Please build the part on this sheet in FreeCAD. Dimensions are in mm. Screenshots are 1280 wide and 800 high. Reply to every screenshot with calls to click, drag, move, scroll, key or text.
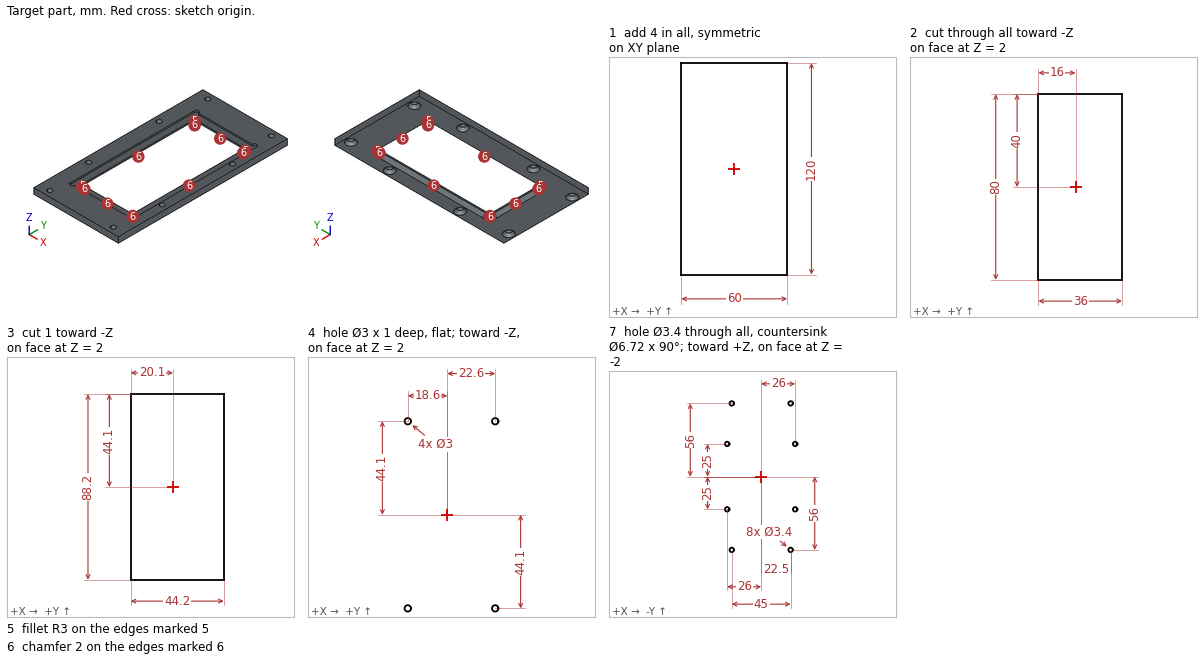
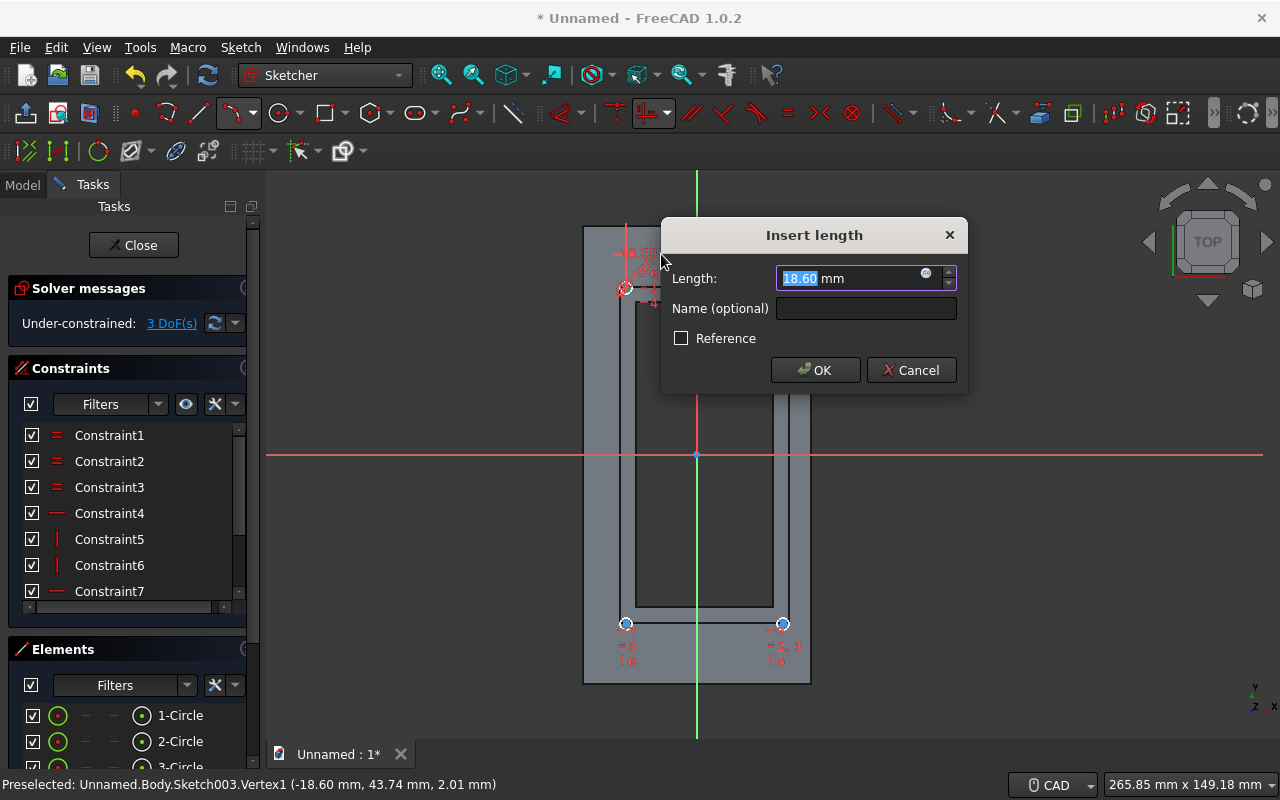
text(18.6)
key(Return)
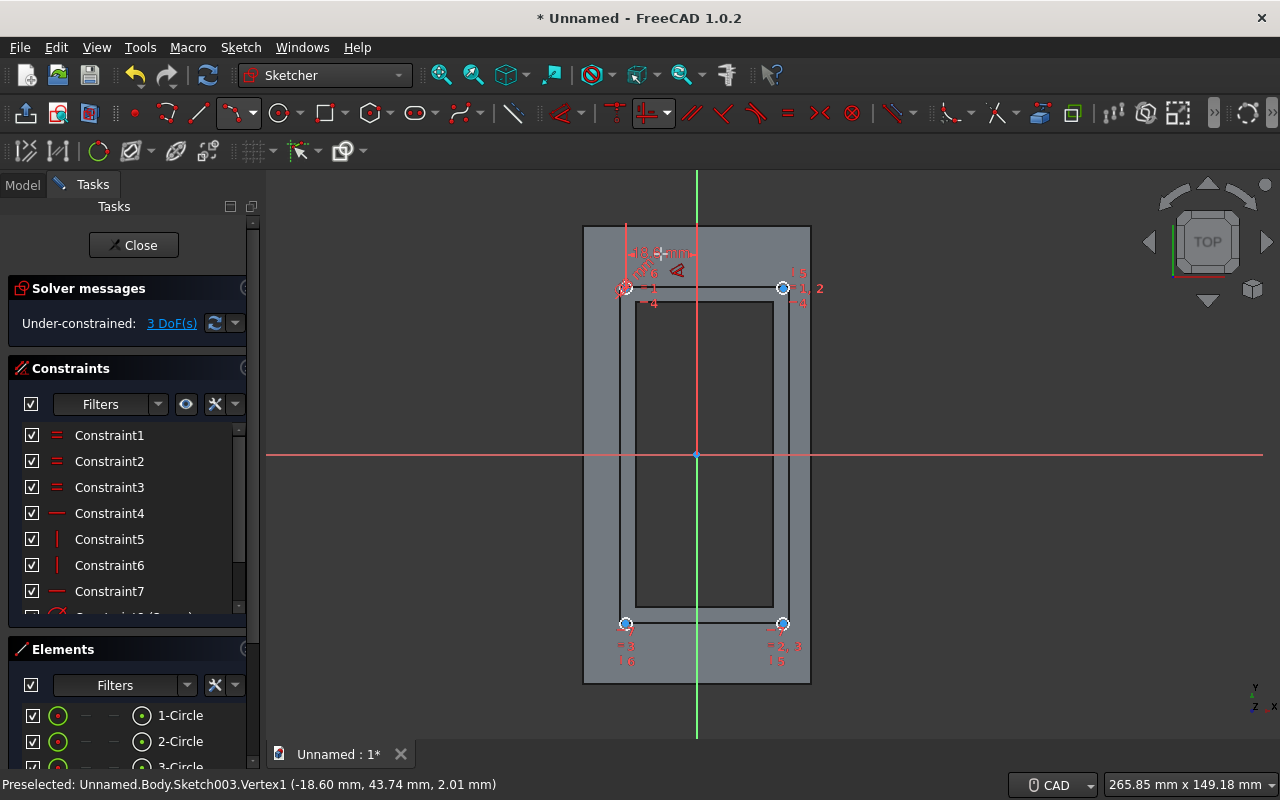
click(626, 288)
click(592, 371)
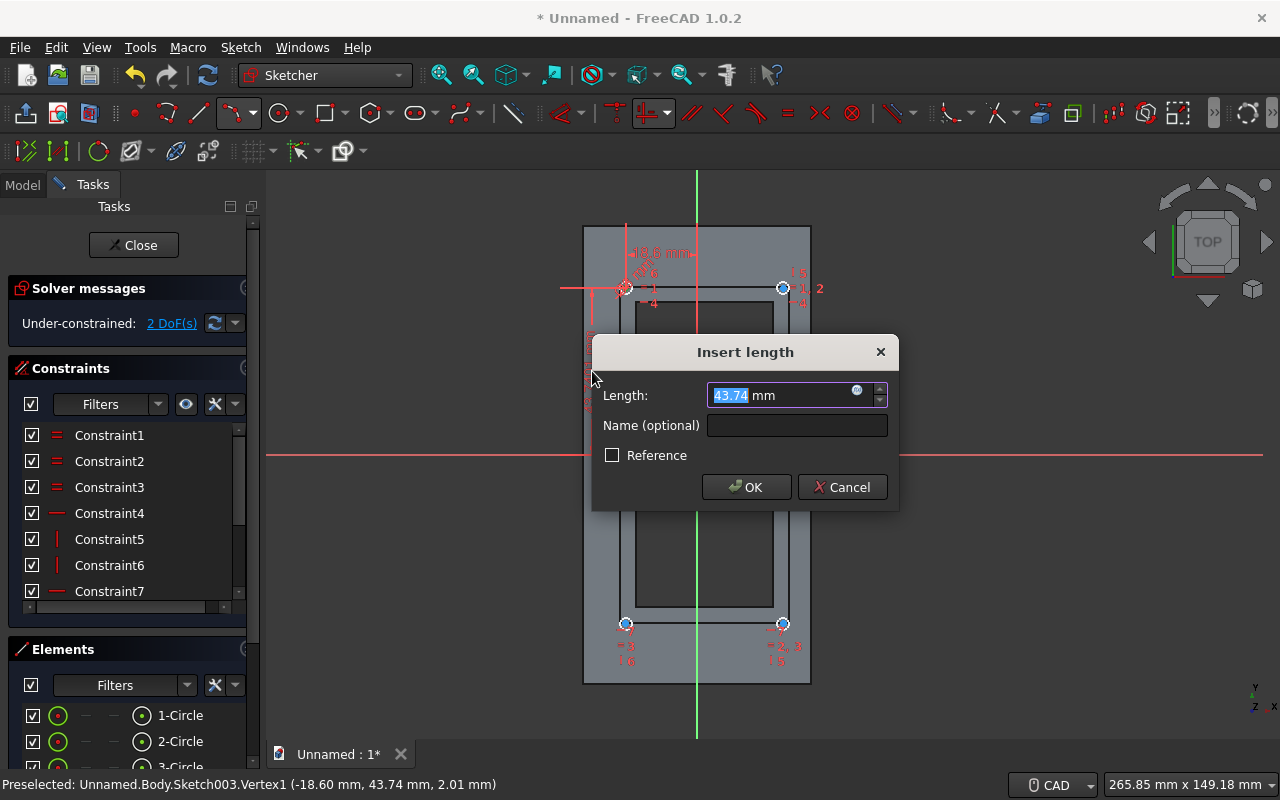
text(44.1)
key(Return)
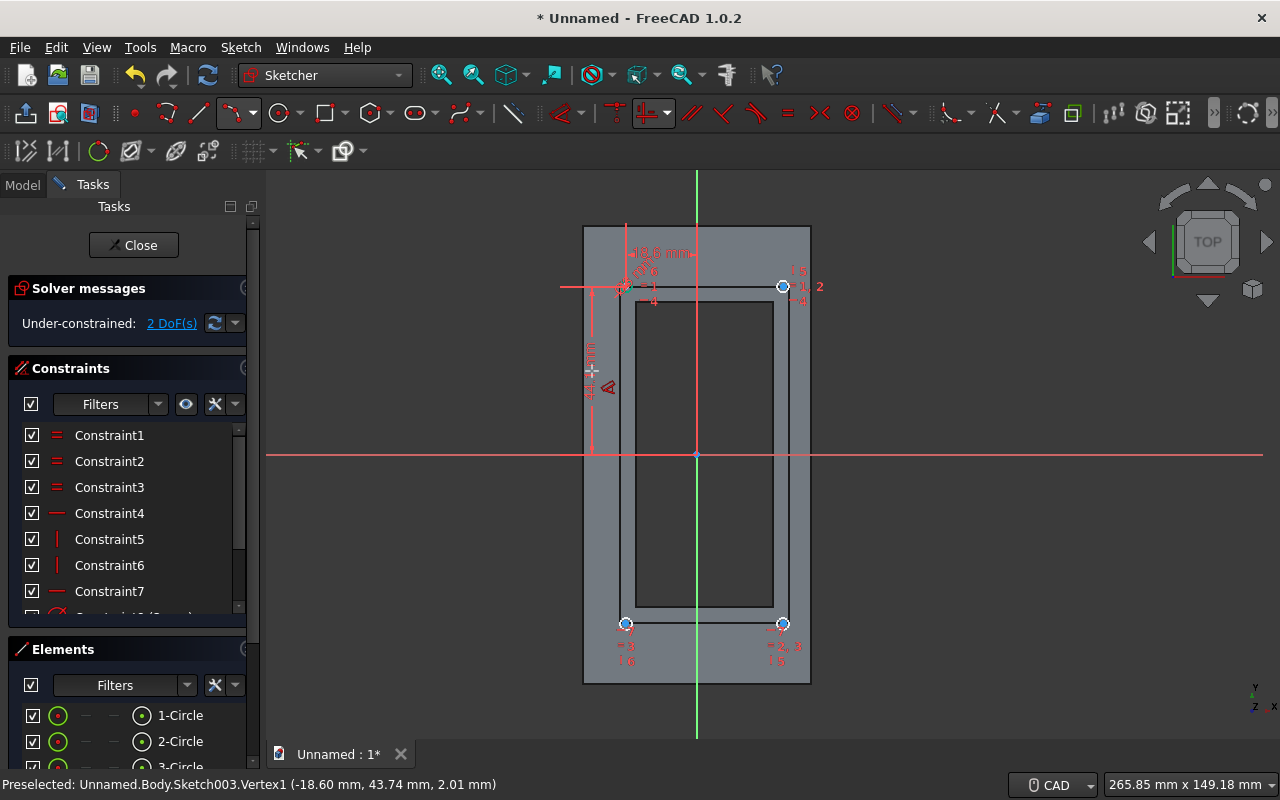
click(783, 287)
click(740, 253)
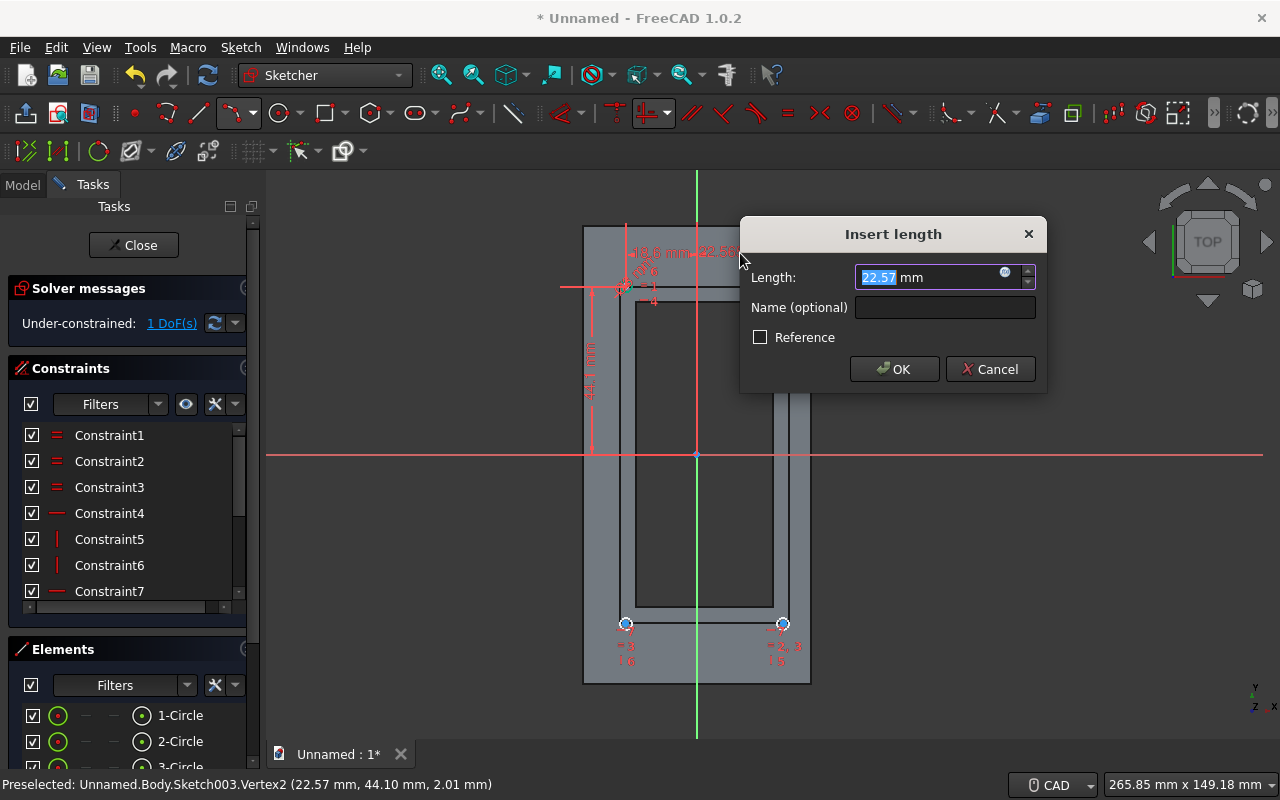
text(22.6)
key(Return)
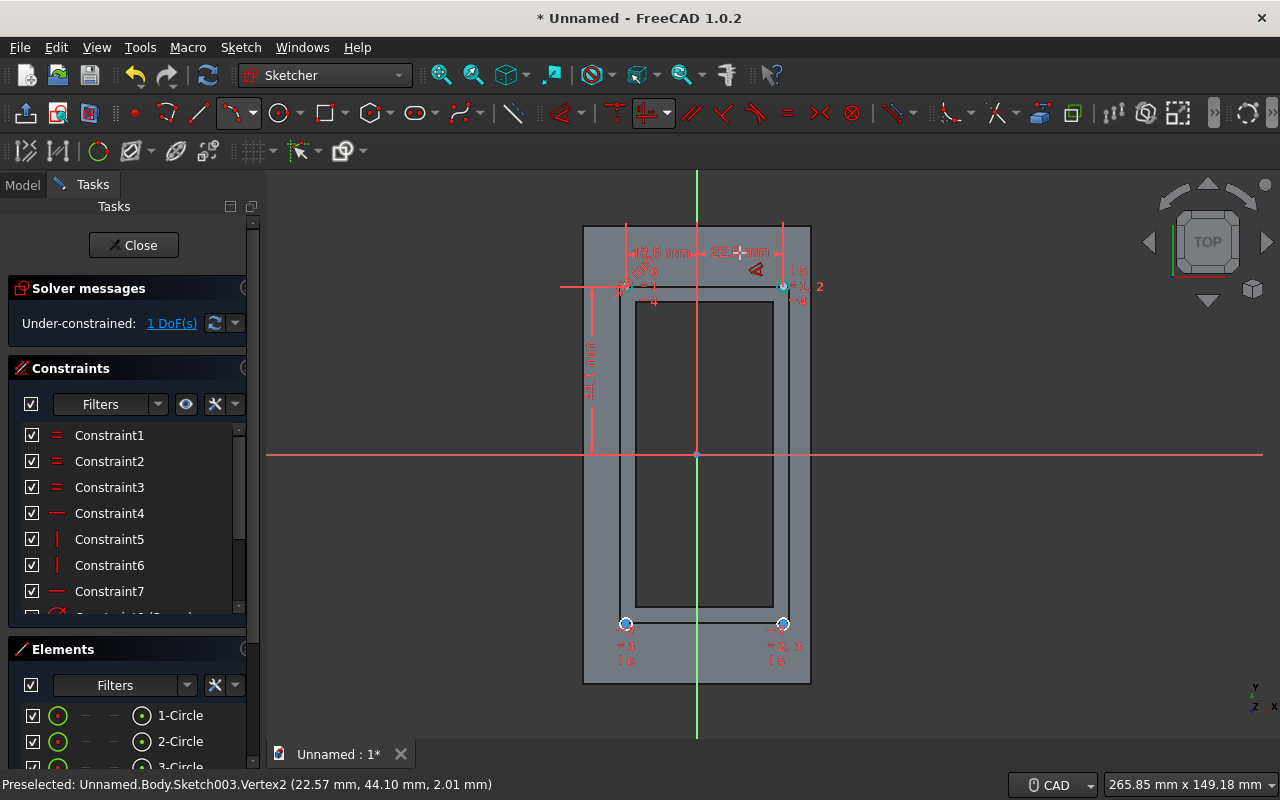
click(783, 624)
click(817, 539)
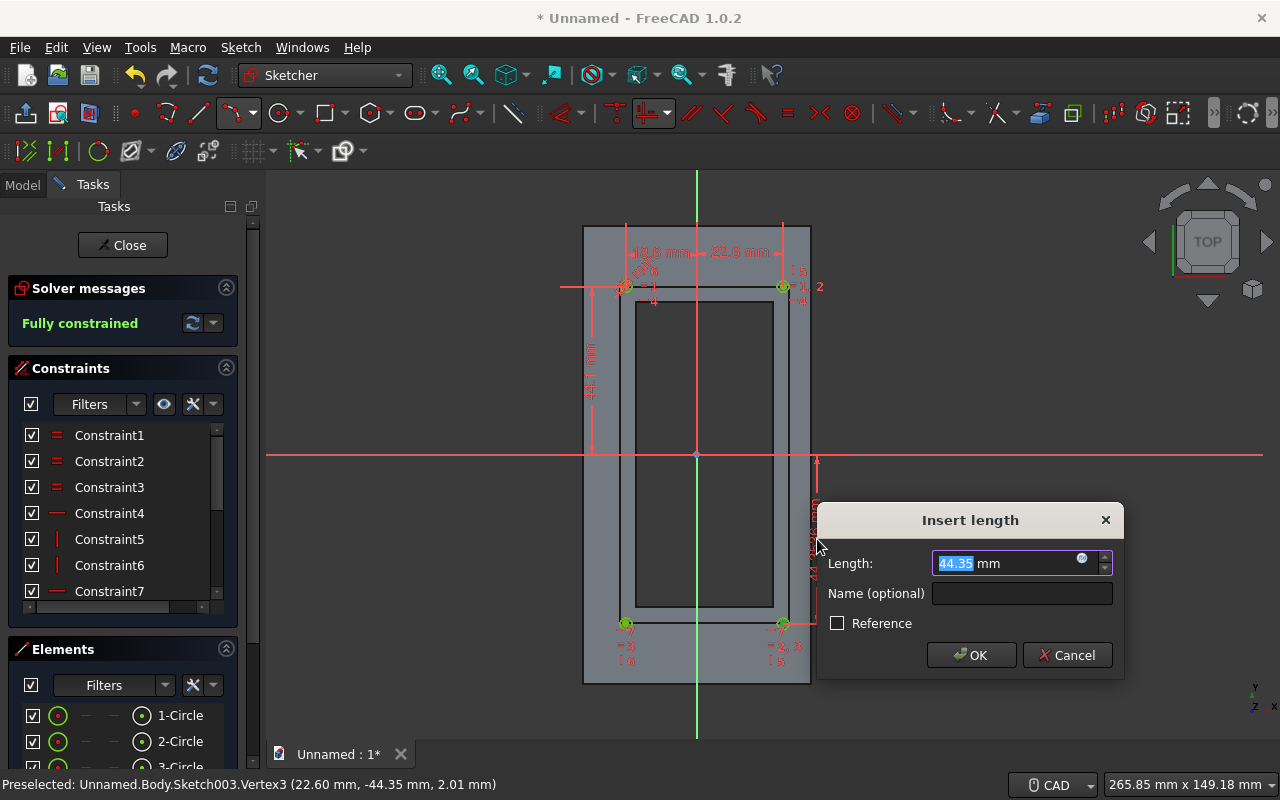
text(44.1)
key(Return)
key(Escape)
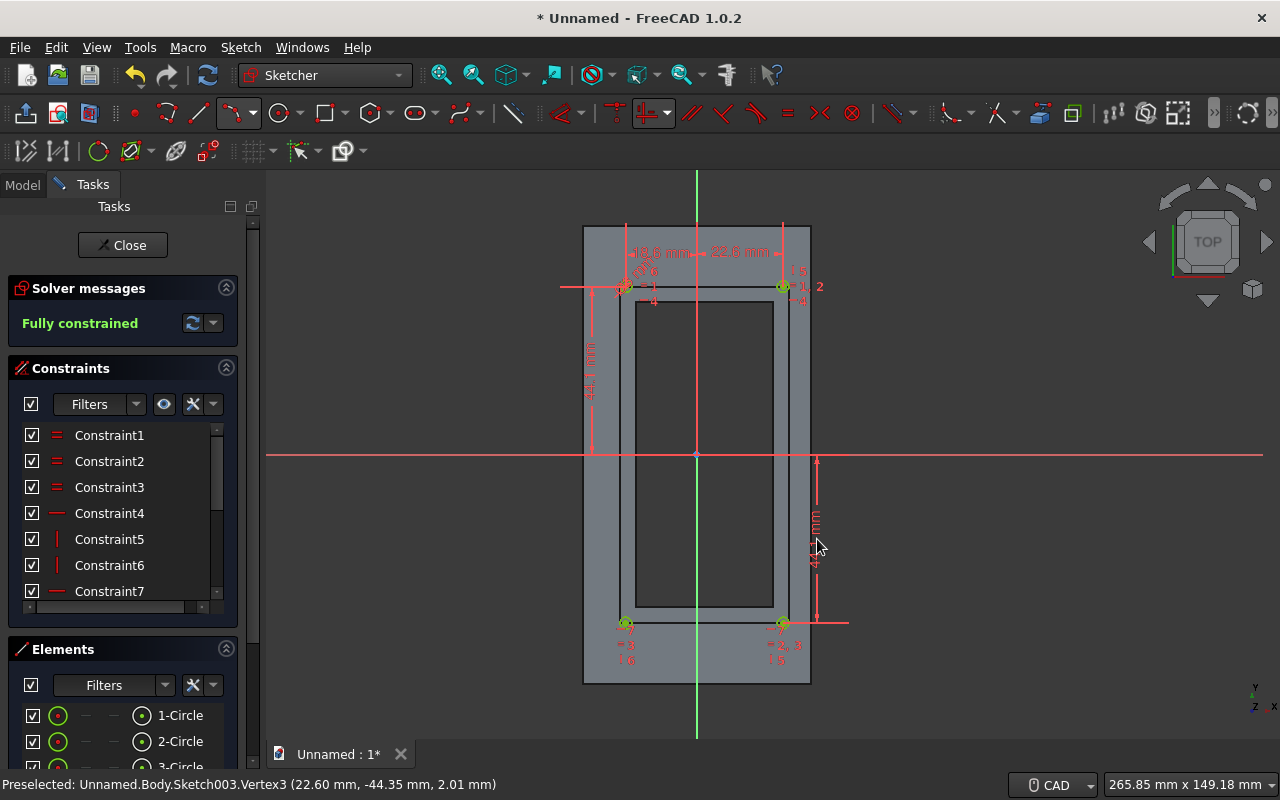
click(123, 245)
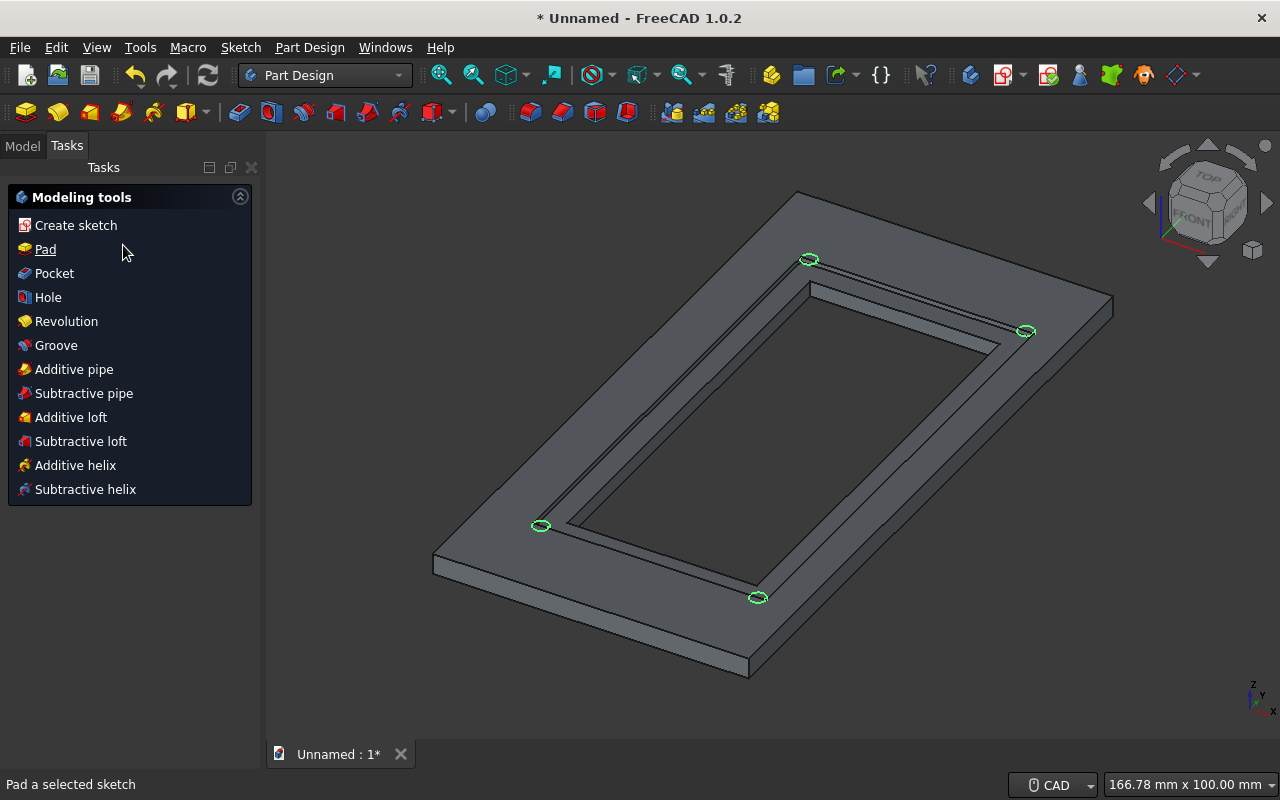
click(272, 112)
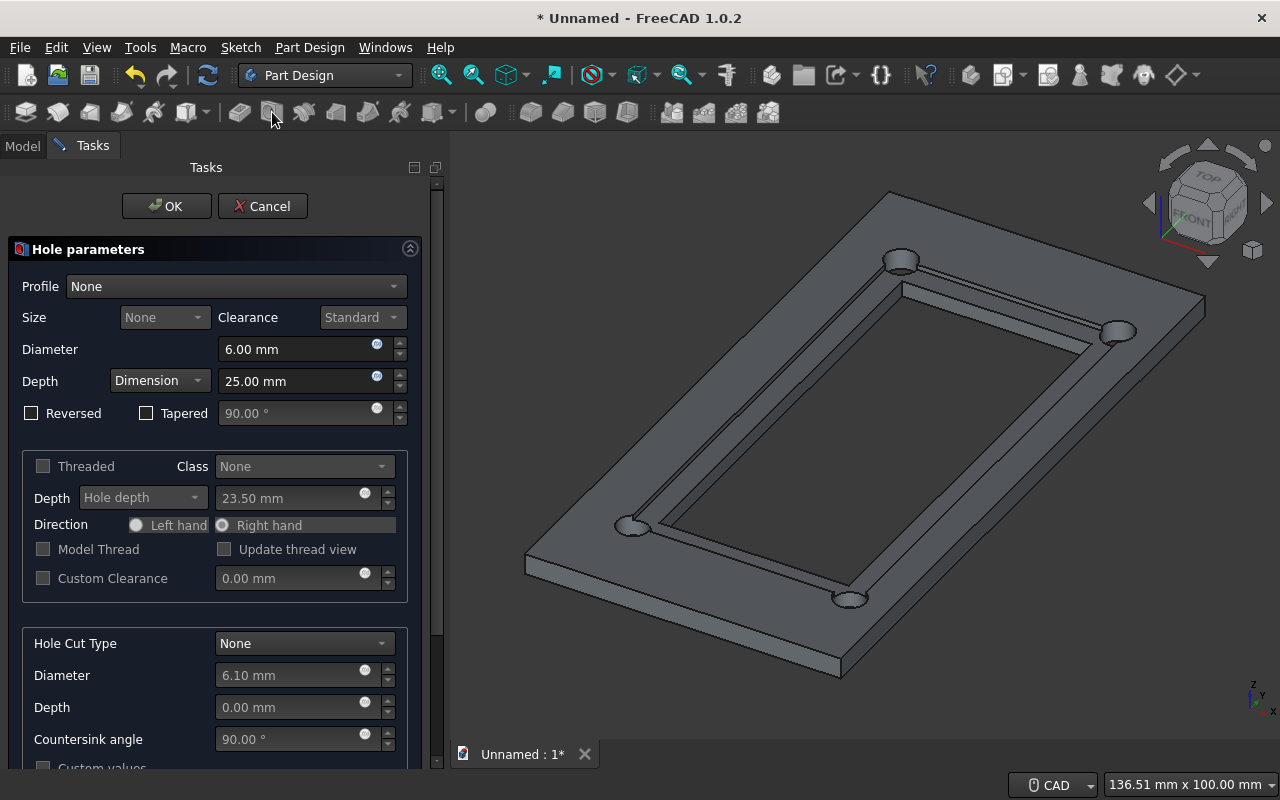
triple_click(305, 349)